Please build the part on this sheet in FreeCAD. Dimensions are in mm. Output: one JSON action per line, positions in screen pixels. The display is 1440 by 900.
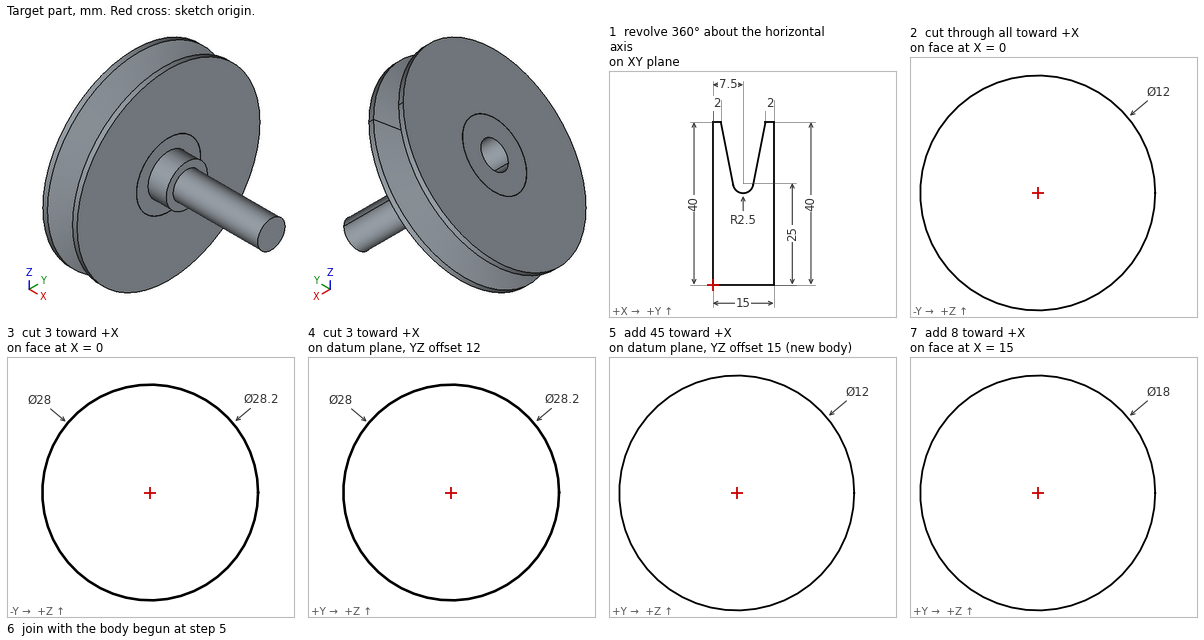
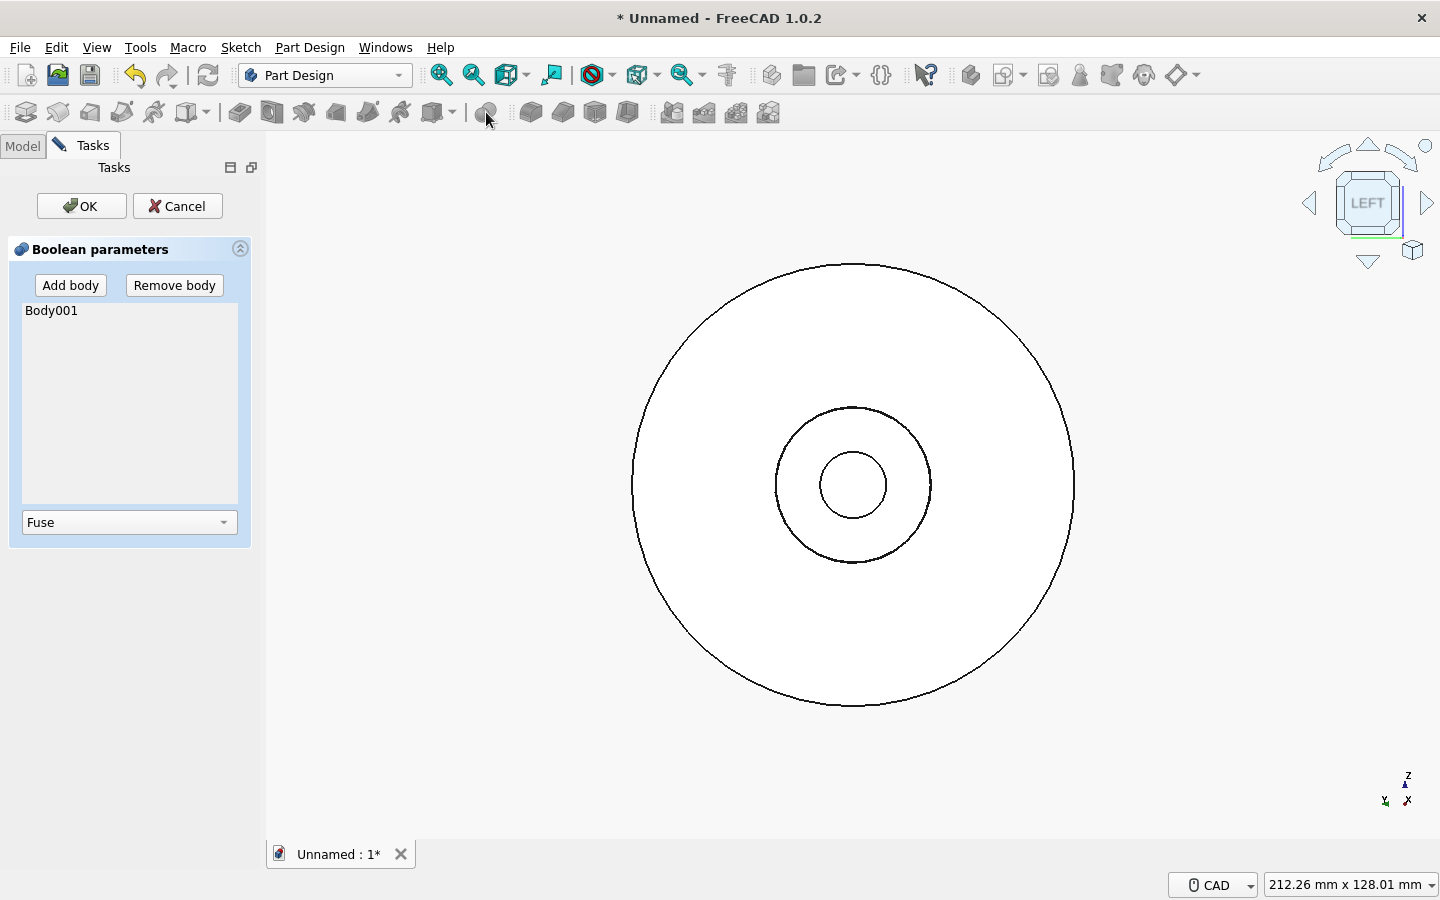
{"action": "left_click", "coordinate": [82, 206]}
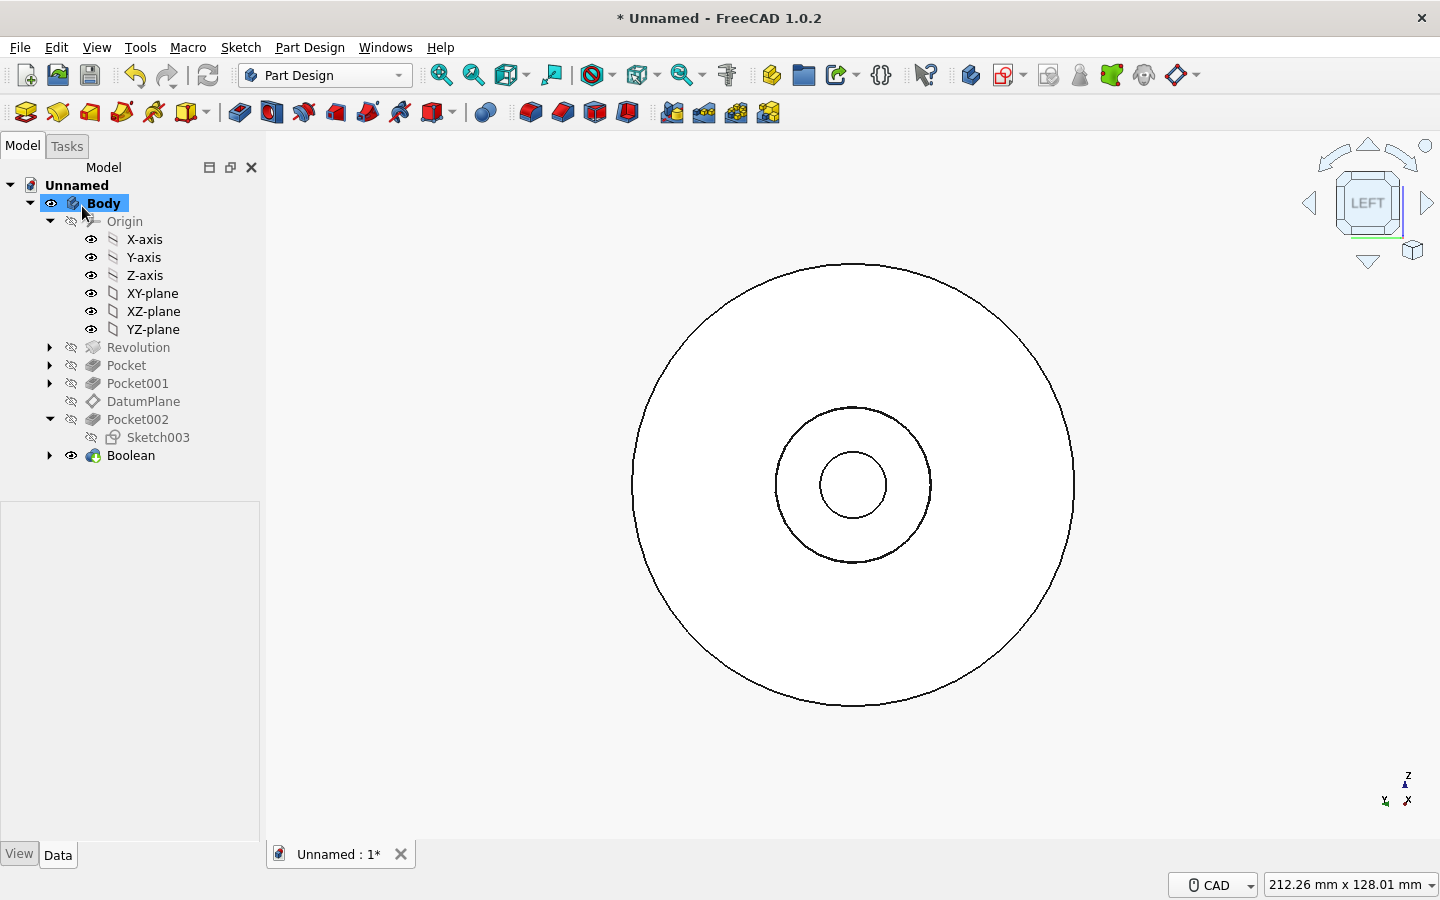
{"action": "key", "text": "0"}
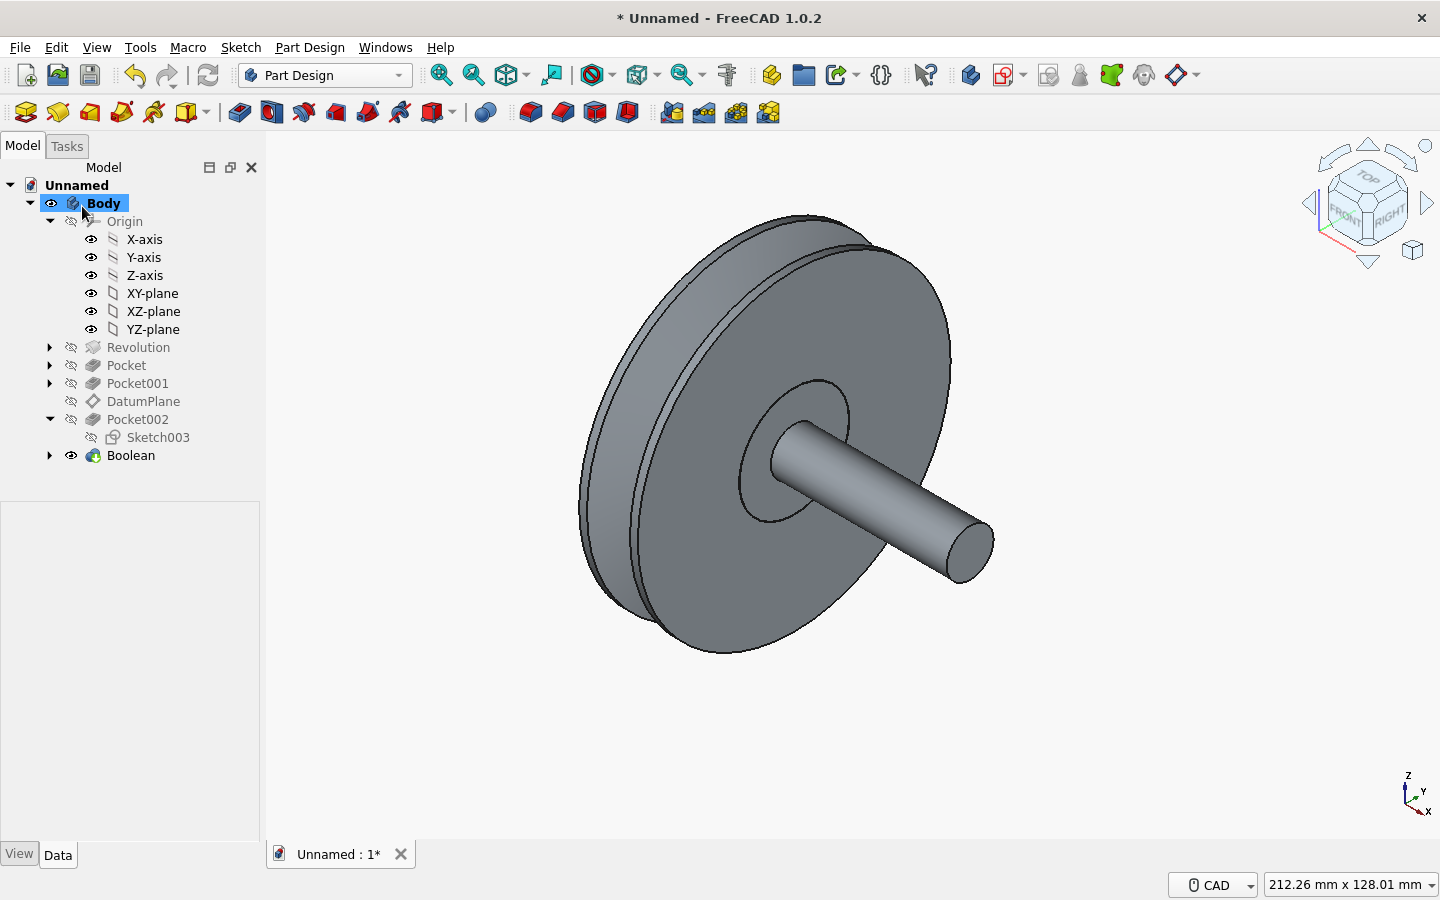
{"action": "left_click", "coordinate": [884, 347]}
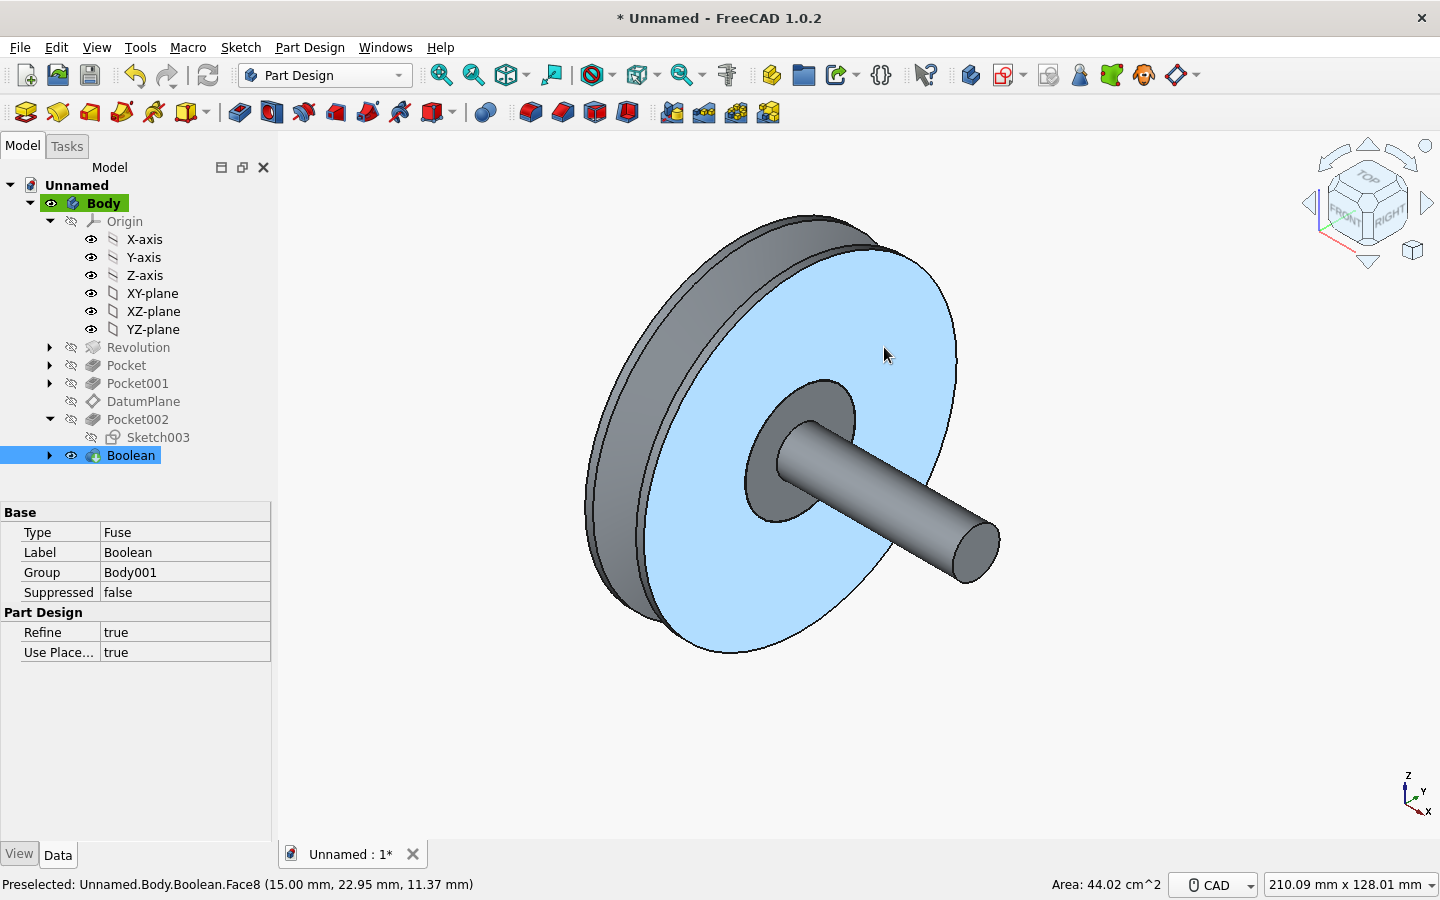
{"action": "left_click", "coordinate": [1004, 76]}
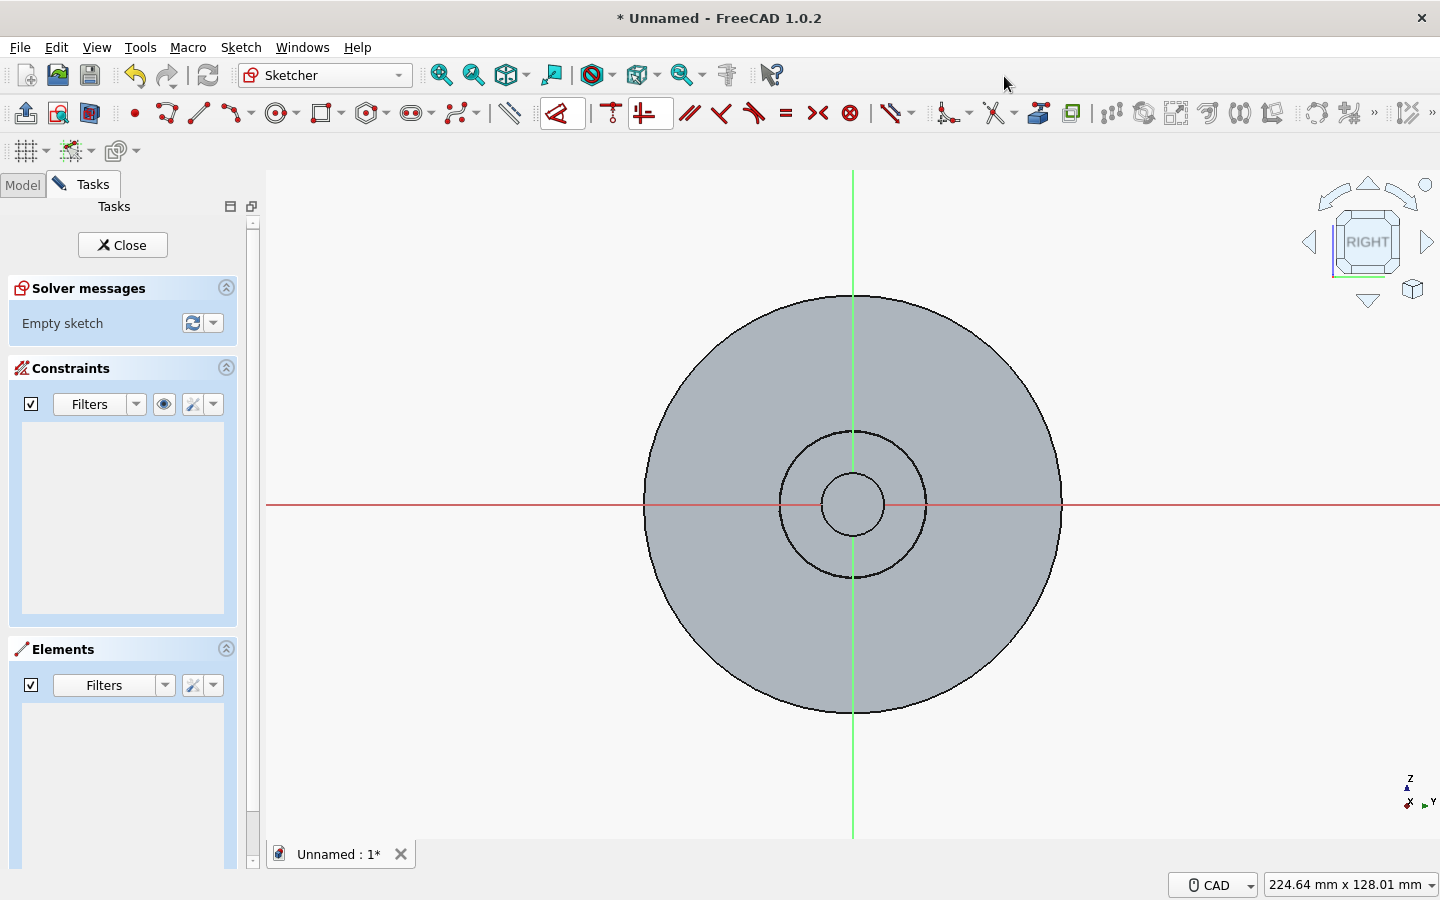
{"action": "left_click", "coordinate": [90, 114]}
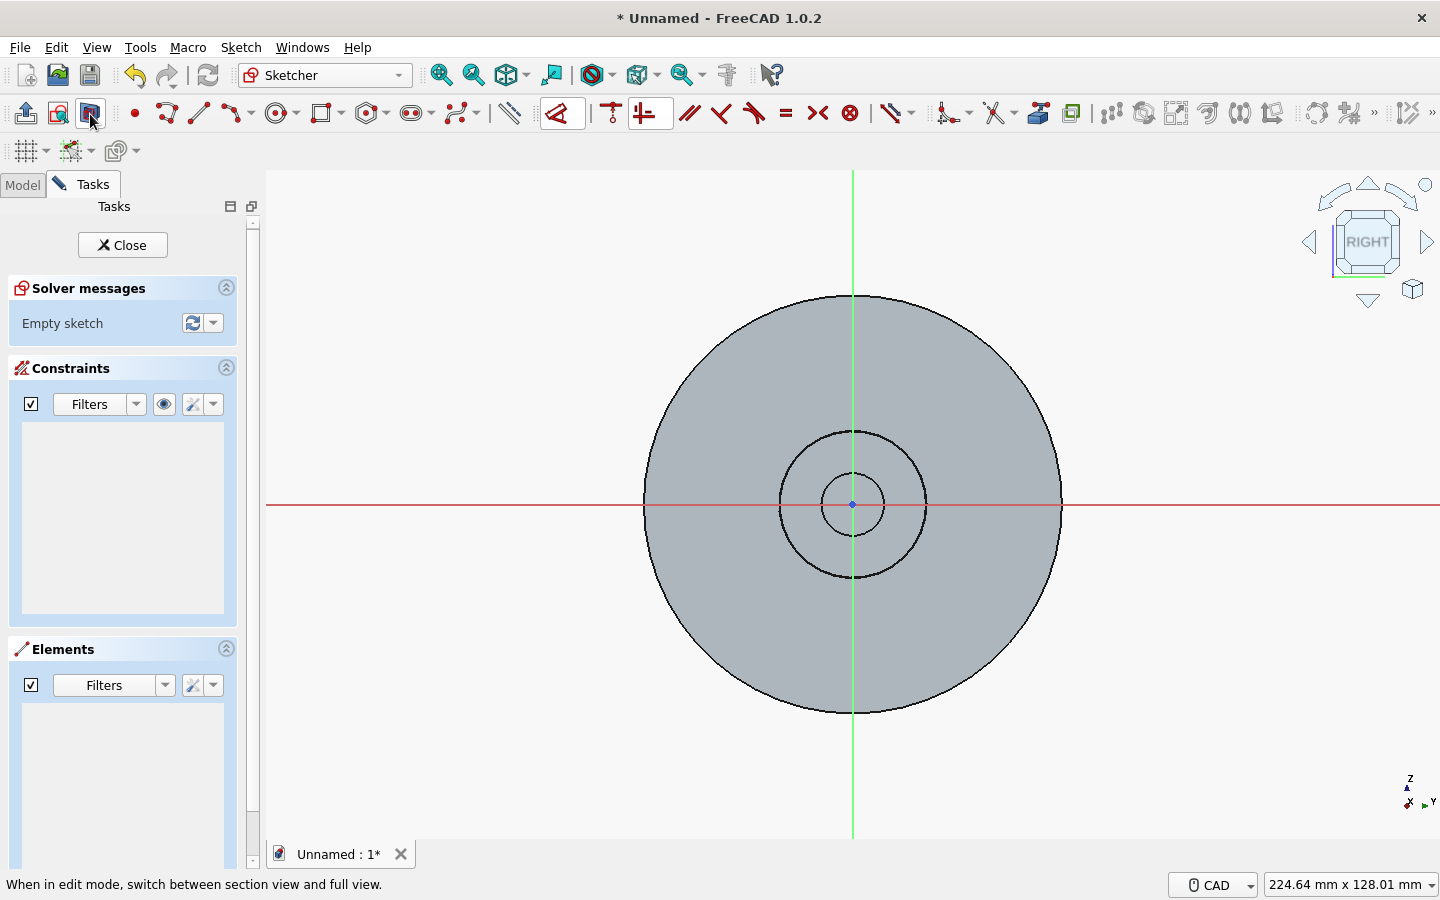
{"action": "scroll", "coordinate": [870, 504], "scroll_direction": "up", "scroll_amount": 8}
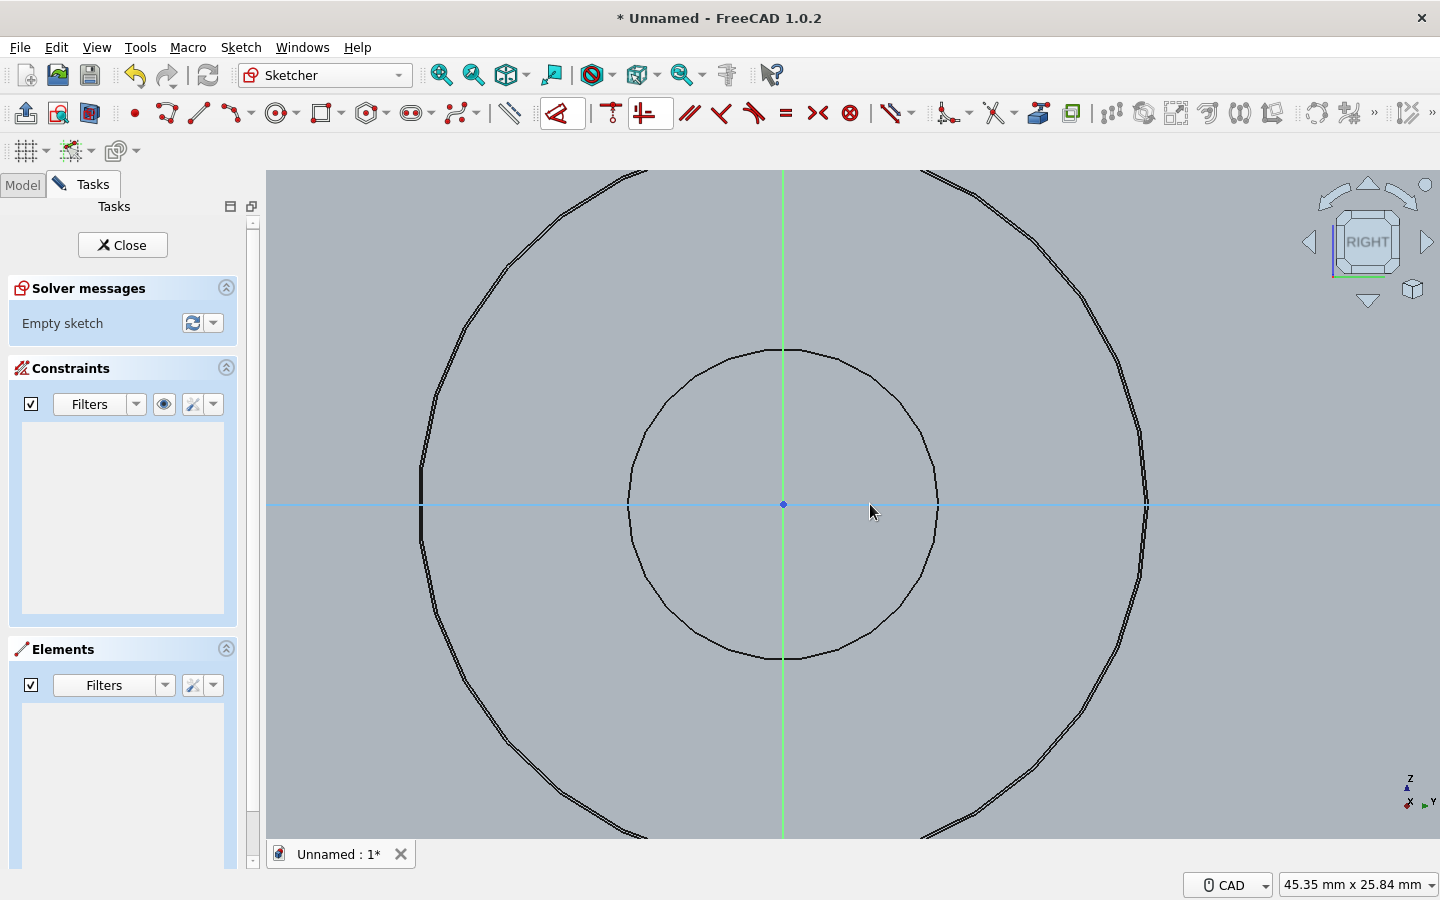
{"action": "left_click", "coordinate": [276, 114]}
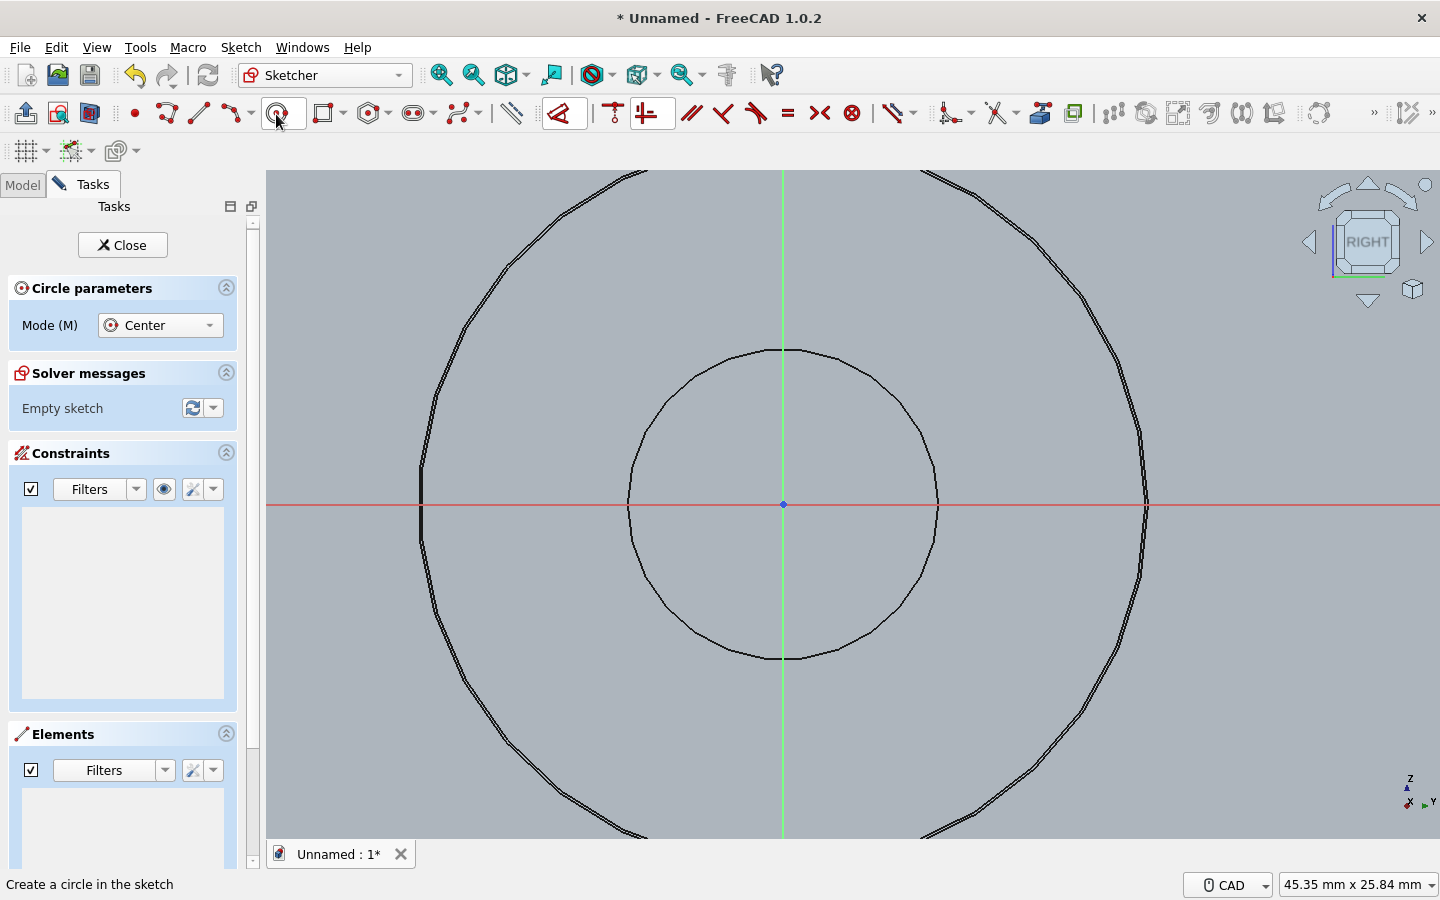
{"action": "left_click", "coordinate": [783, 504]}
{"action": "mouse_move", "coordinate": [948, 340]}